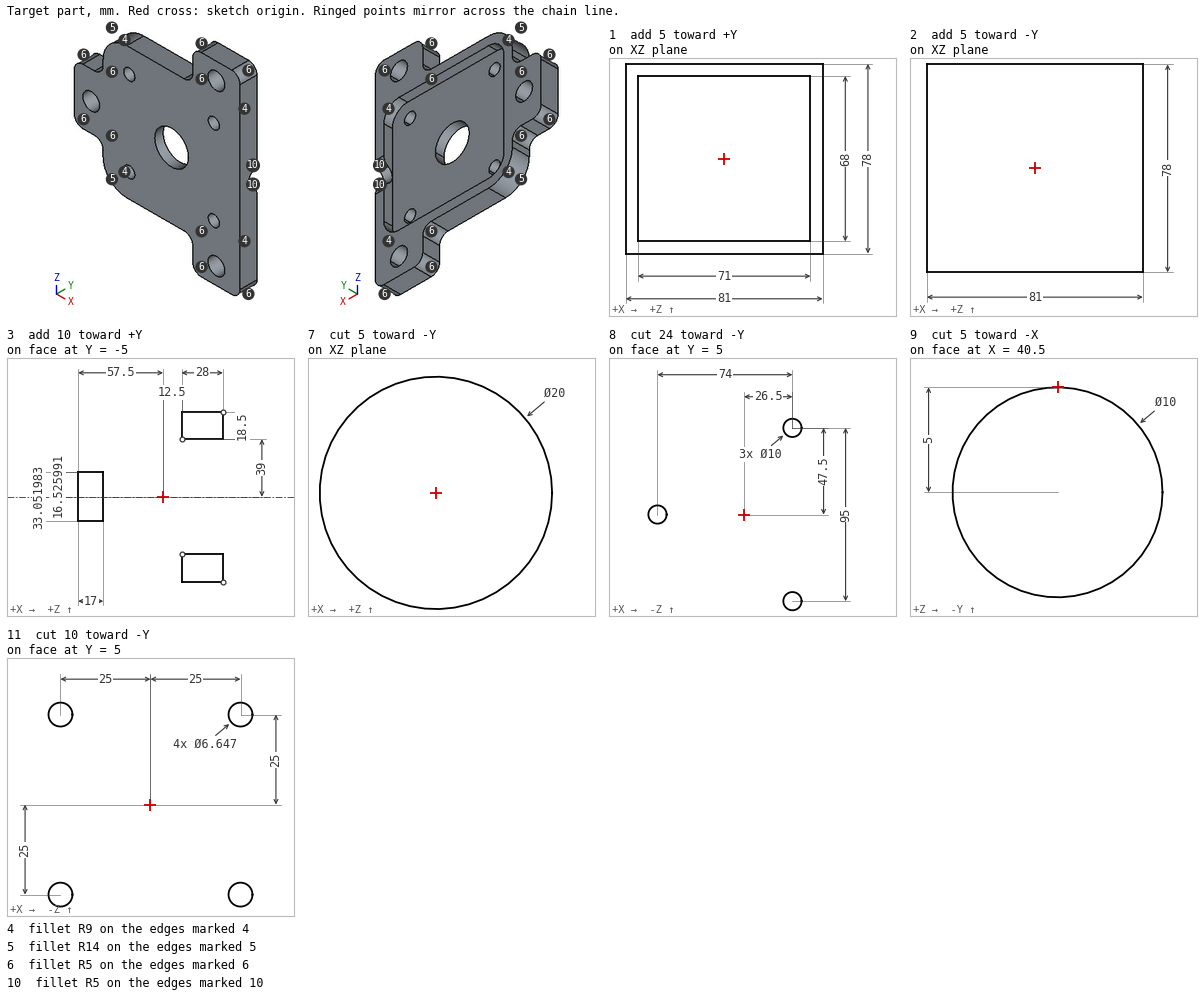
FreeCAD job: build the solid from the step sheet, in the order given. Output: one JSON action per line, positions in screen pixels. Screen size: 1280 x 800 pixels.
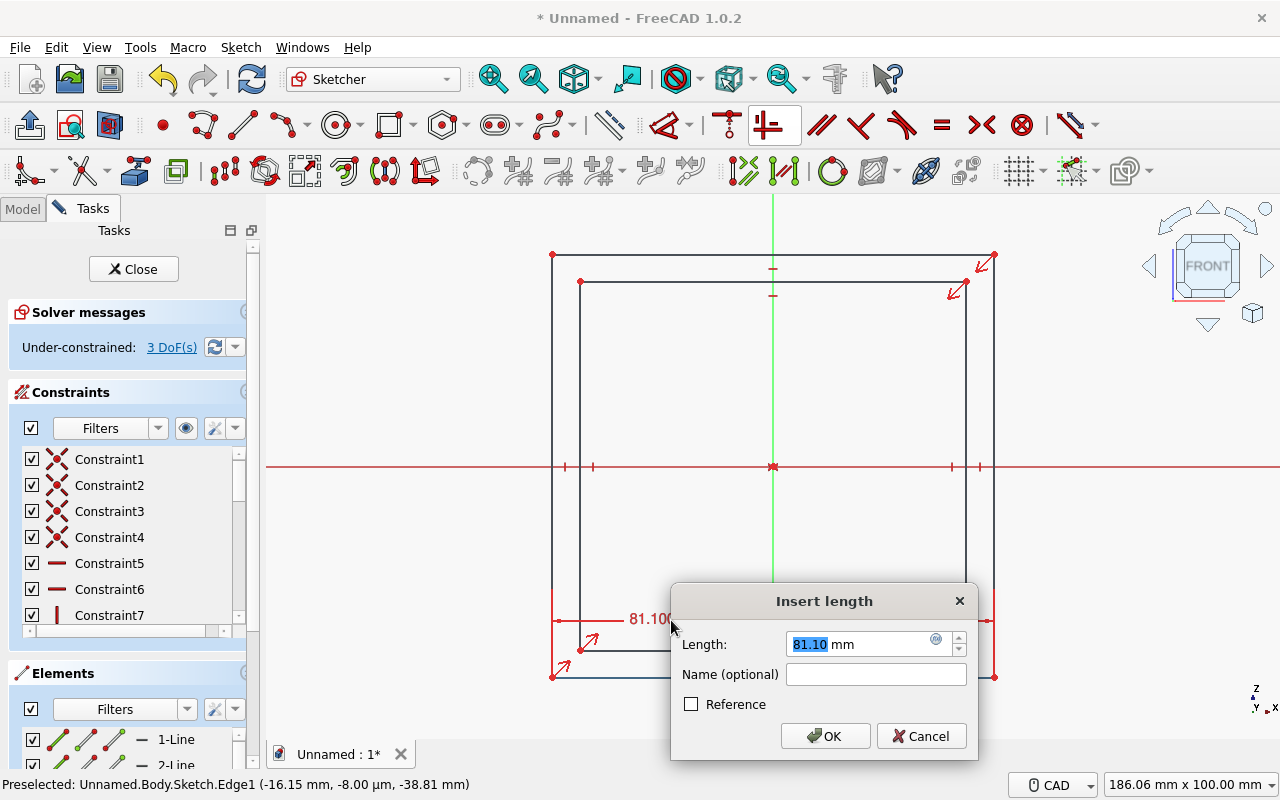
{"action": "type", "text": "81"}
{"action": "key", "text": "Return"}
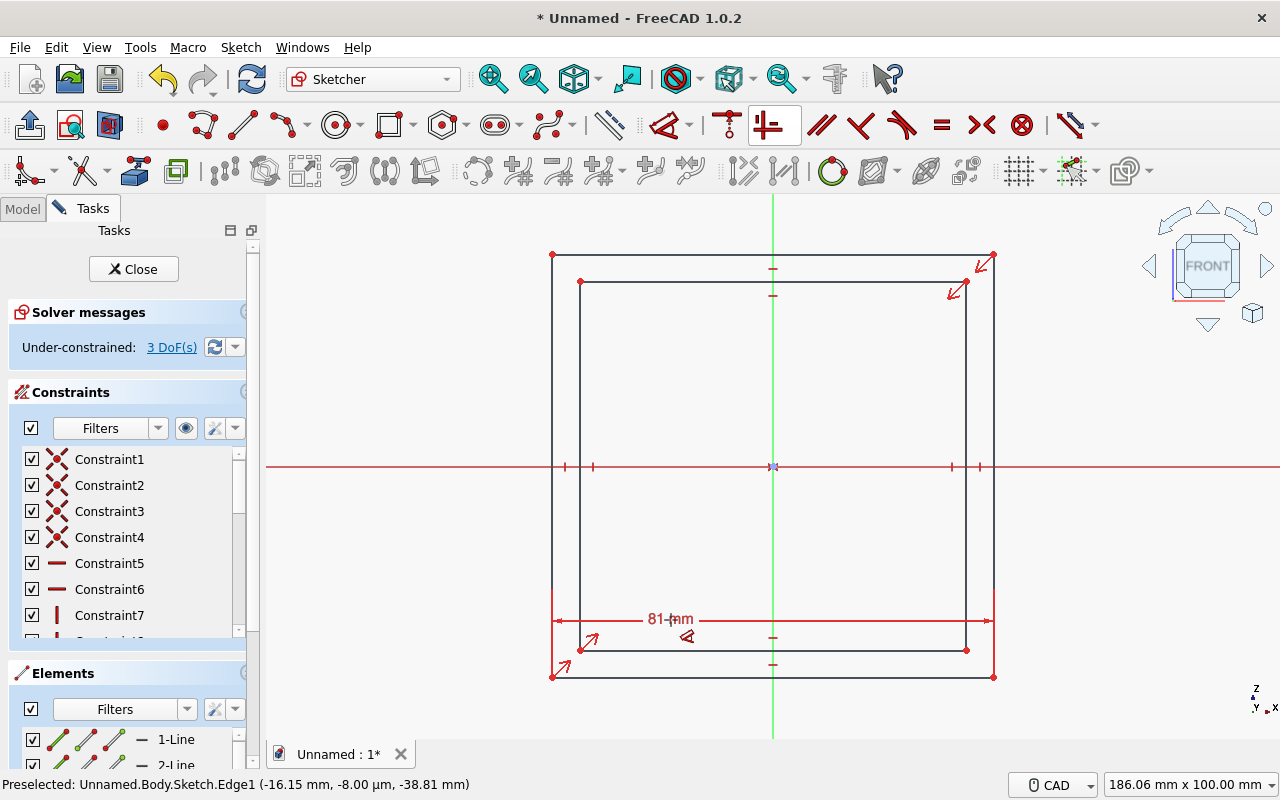
{"action": "left_click", "coordinate": [994, 551]}
{"action": "left_click", "coordinate": [1028, 369]}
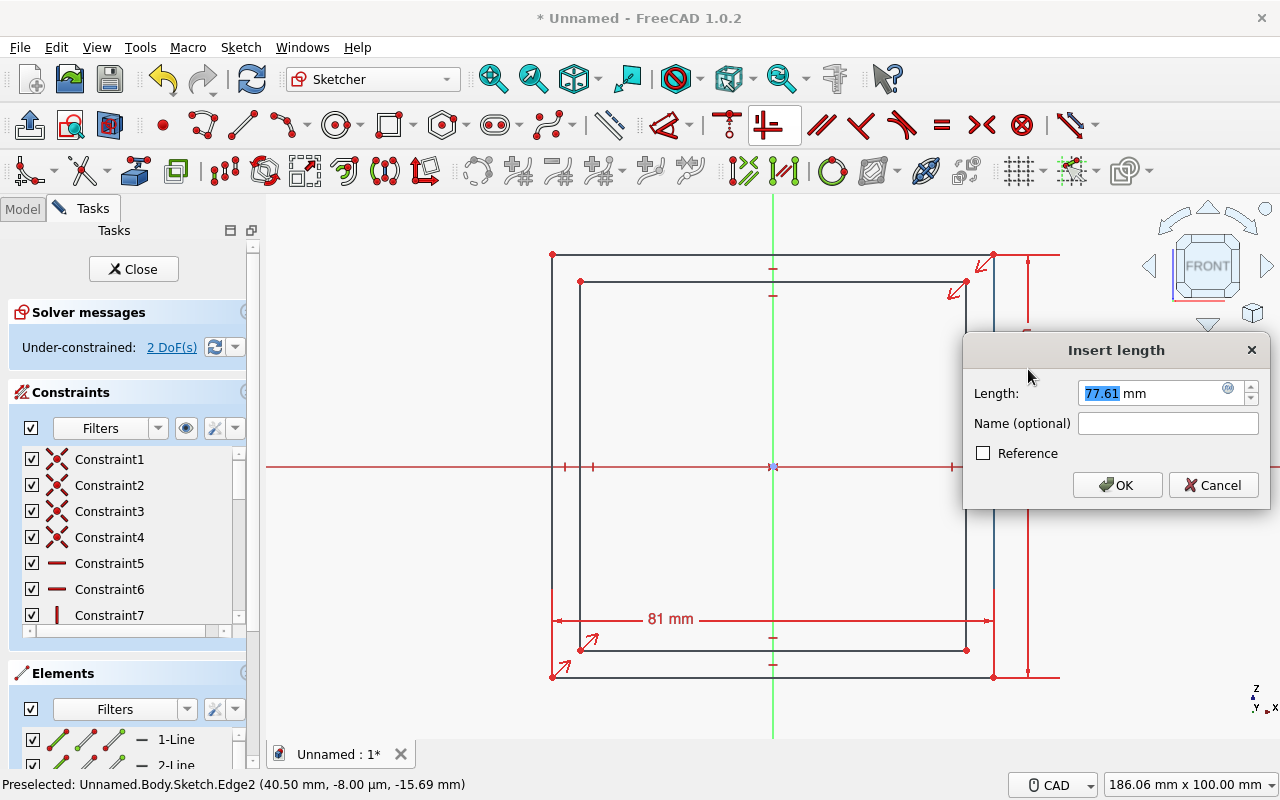
{"action": "type", "text": "78"}
{"action": "key", "text": "Return"}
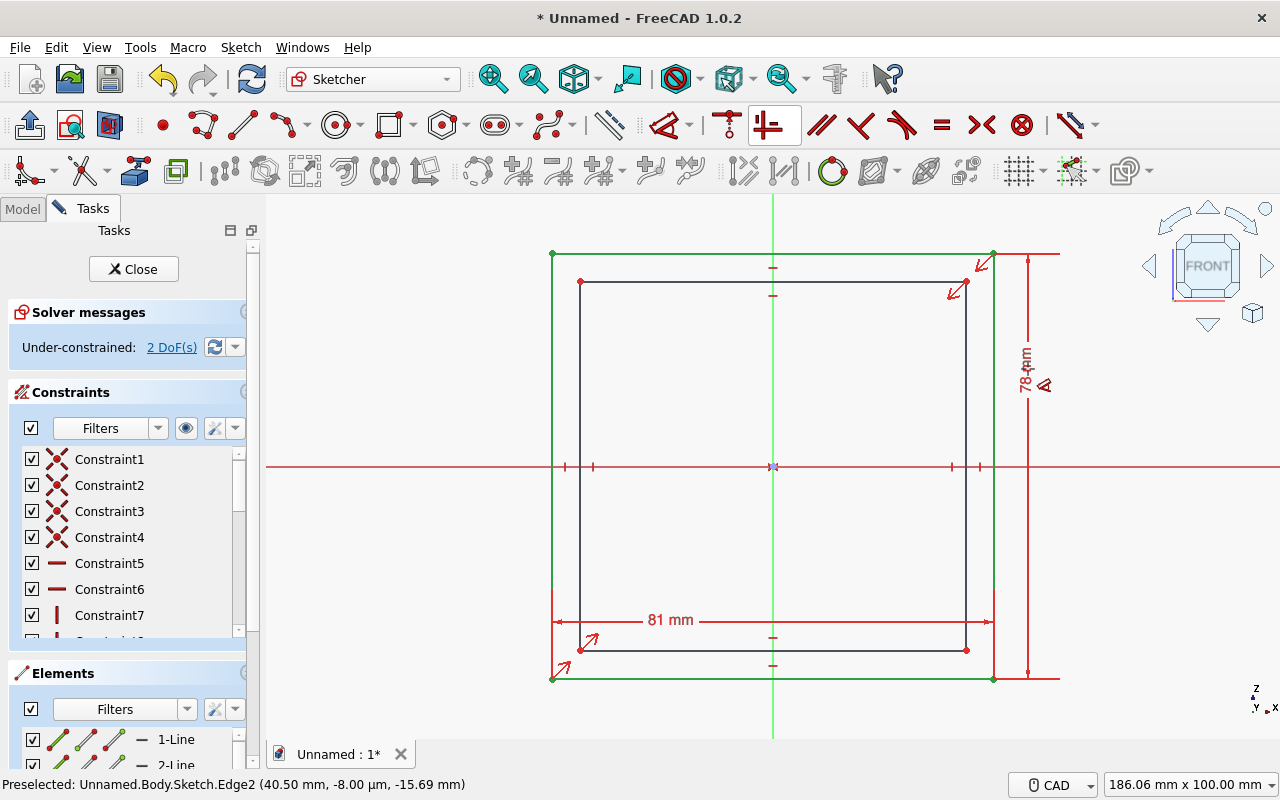
{"action": "left_click", "coordinate": [696, 651]}
{"action": "left_click", "coordinate": [862, 617]}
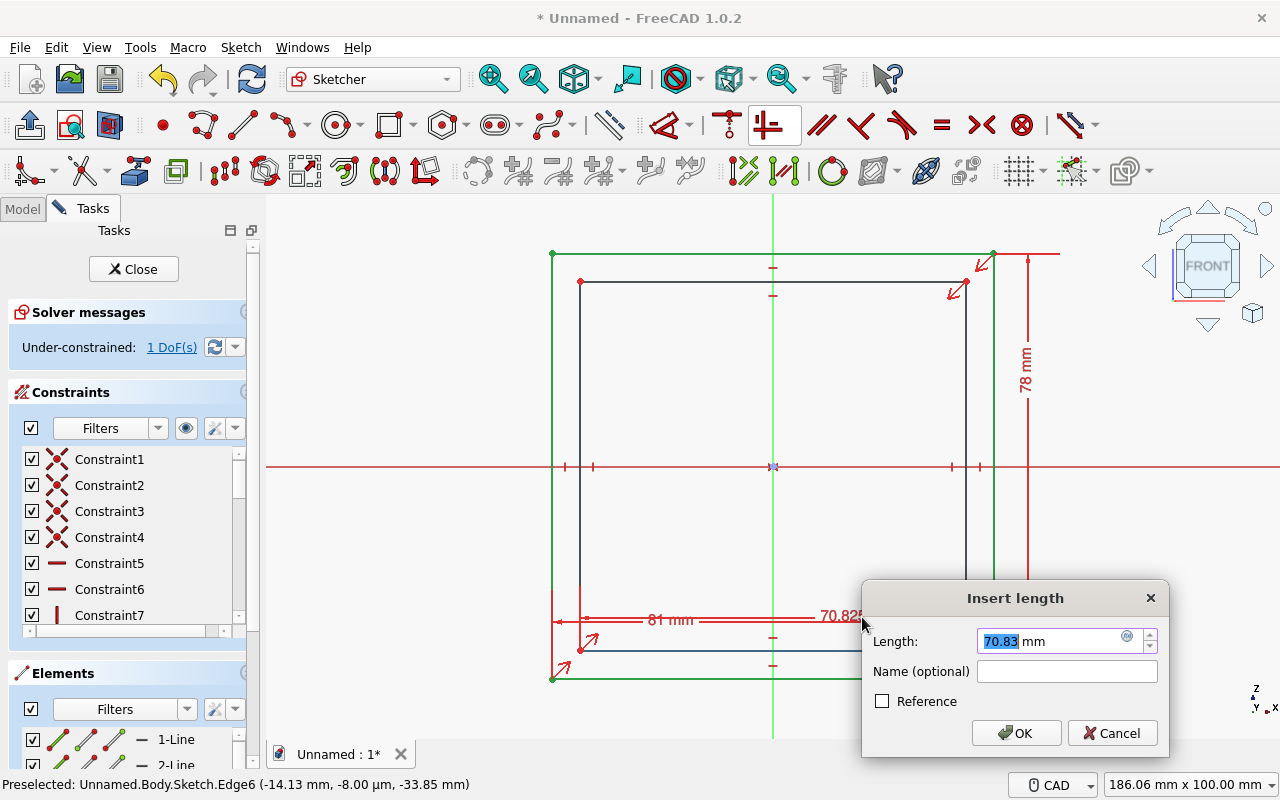
{"action": "type", "text": "71"}
{"action": "key", "text": "Return"}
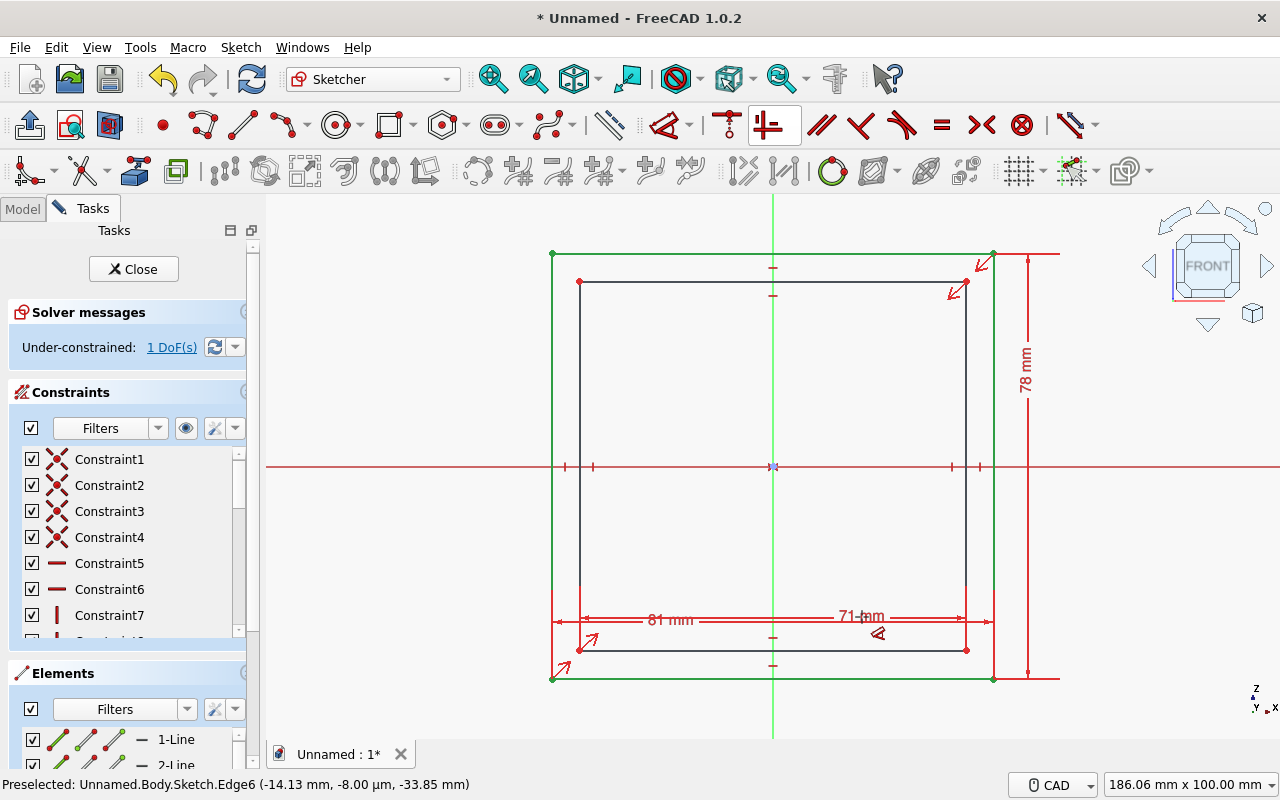
{"action": "left_click", "coordinate": [966, 540]}
{"action": "left_click", "coordinate": [932, 382]}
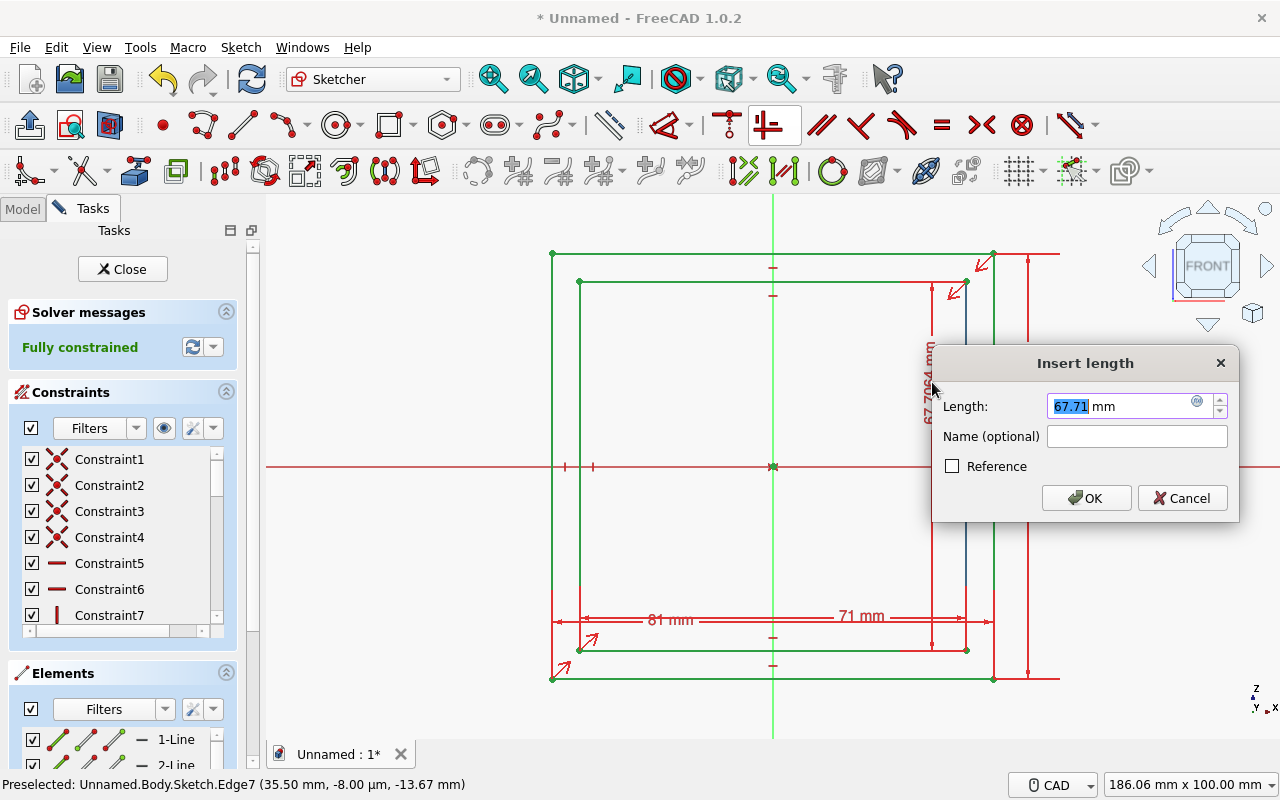
{"action": "type", "text": "68"}
{"action": "key", "text": "Return"}
{"action": "key", "text": "Escape"}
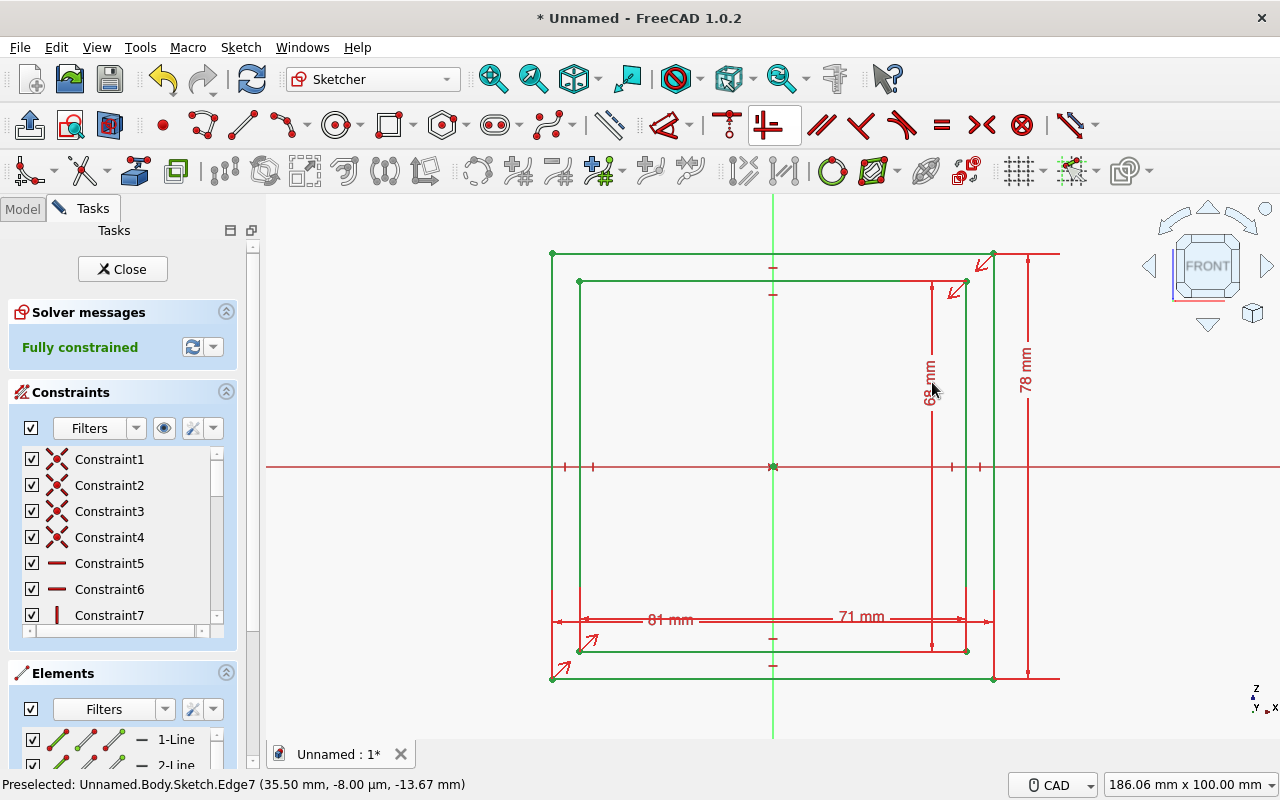
{"action": "left_click", "coordinate": [123, 269]}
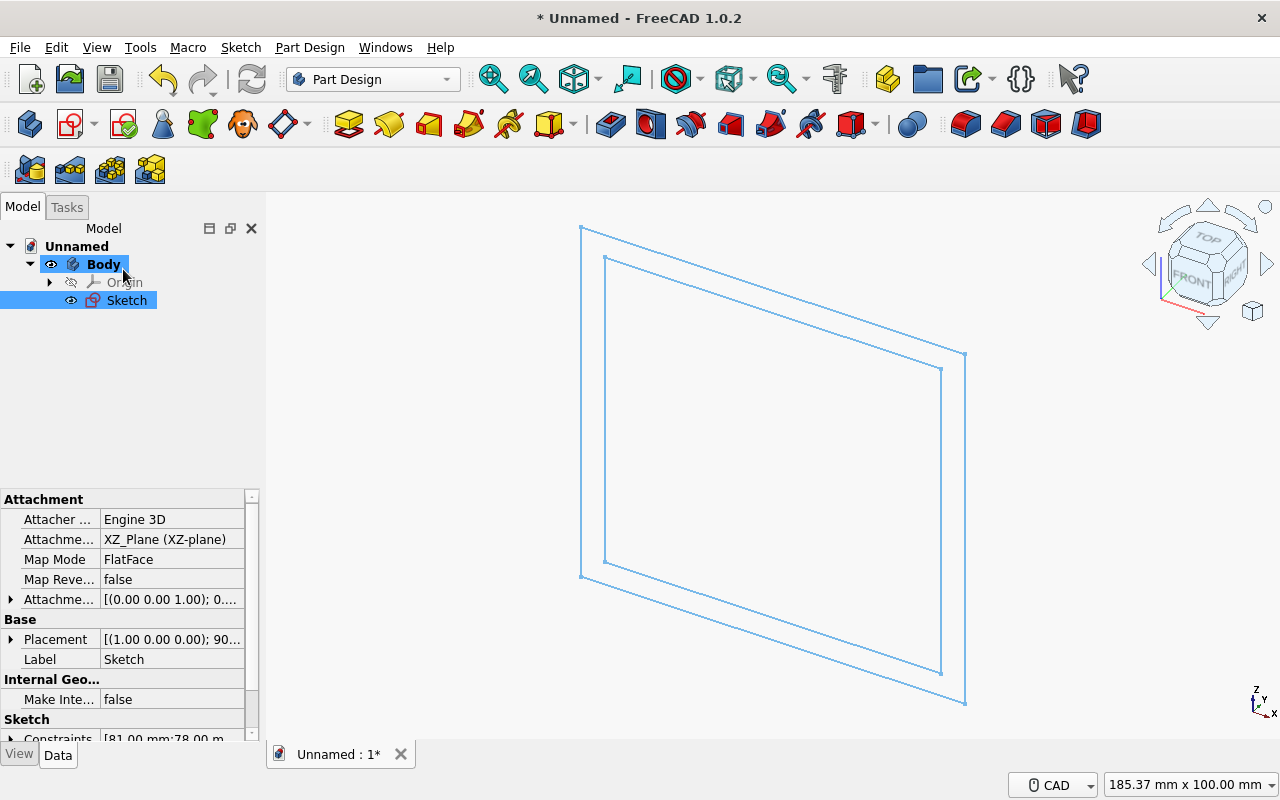
{"action": "left_click", "coordinate": [350, 124]}